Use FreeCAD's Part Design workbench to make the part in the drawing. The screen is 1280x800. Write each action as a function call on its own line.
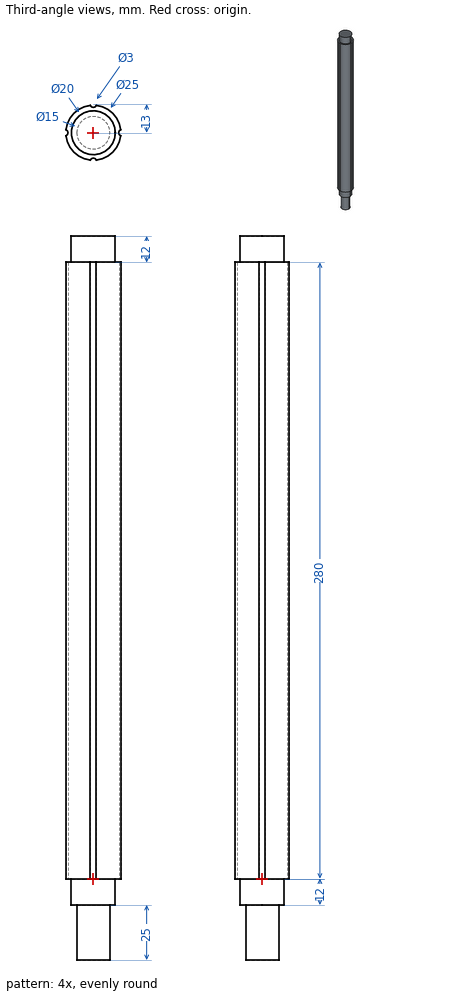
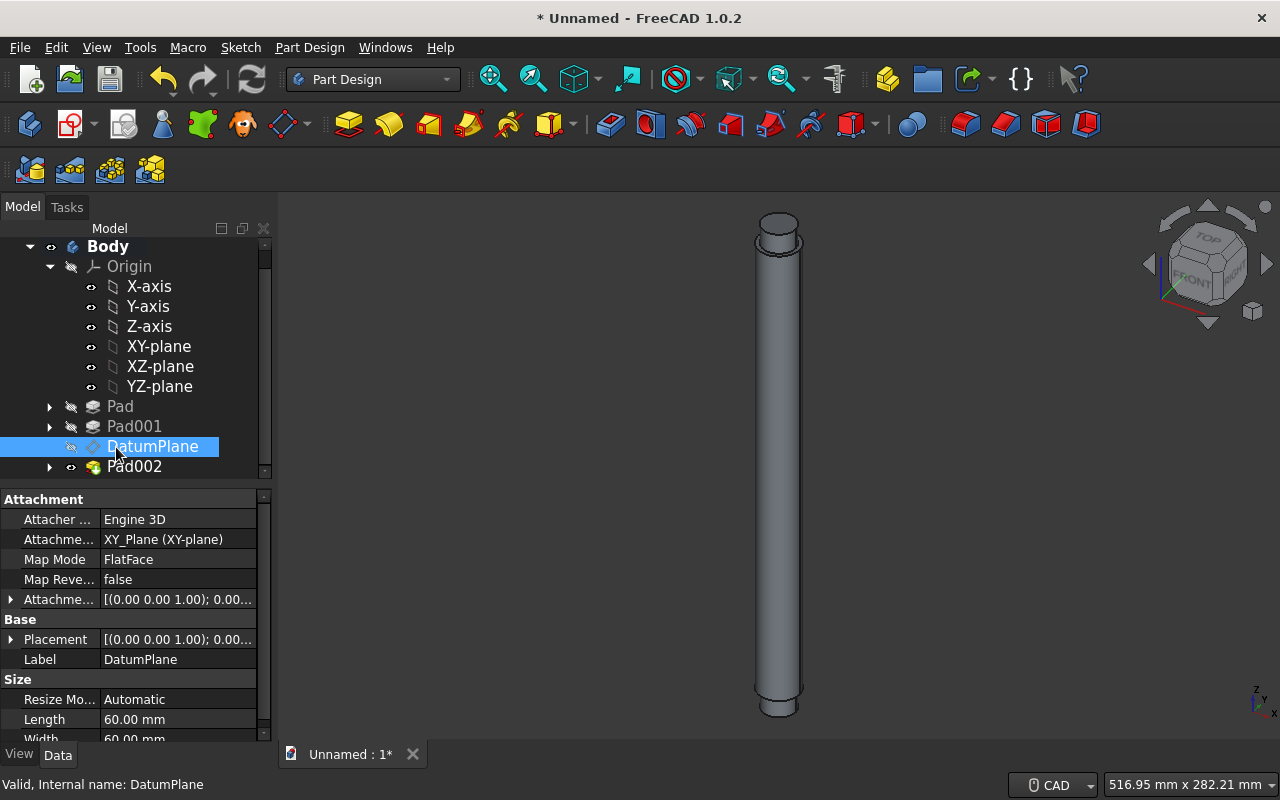
key(5)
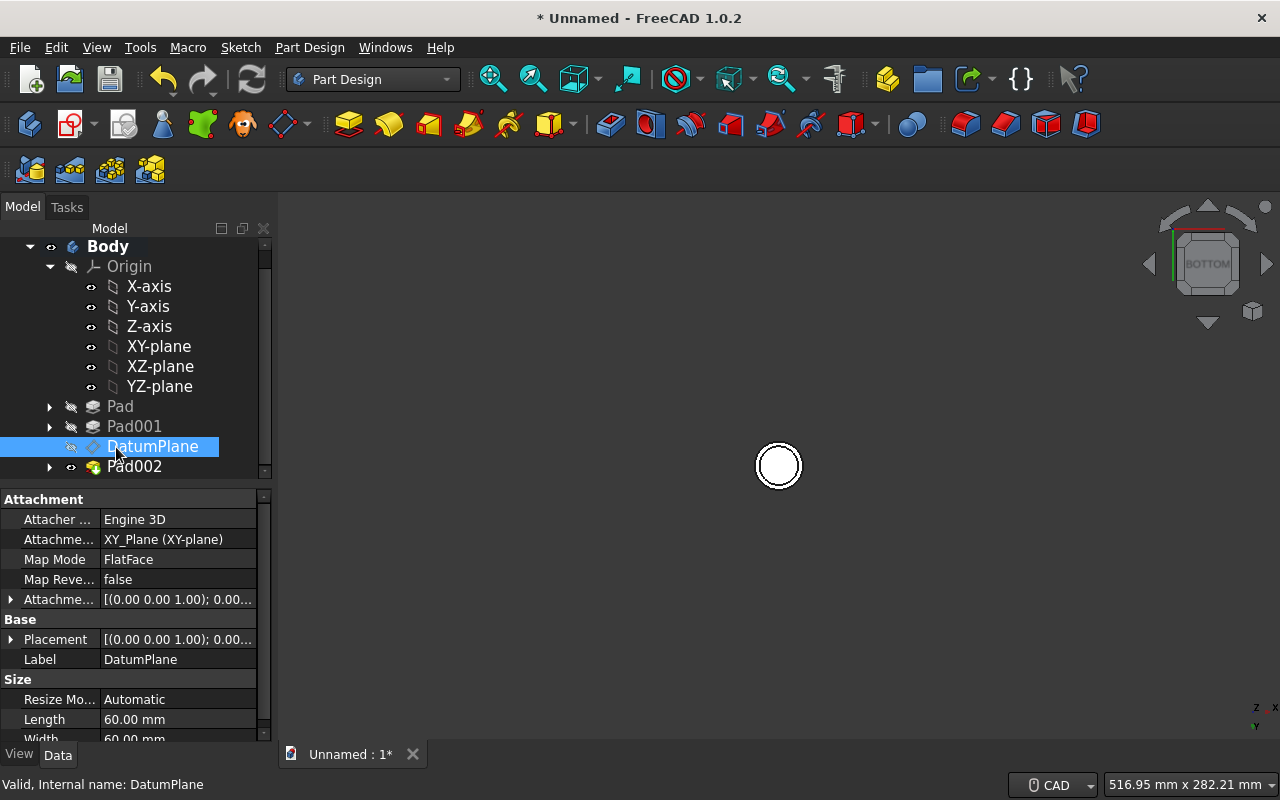
key(v)
key(f)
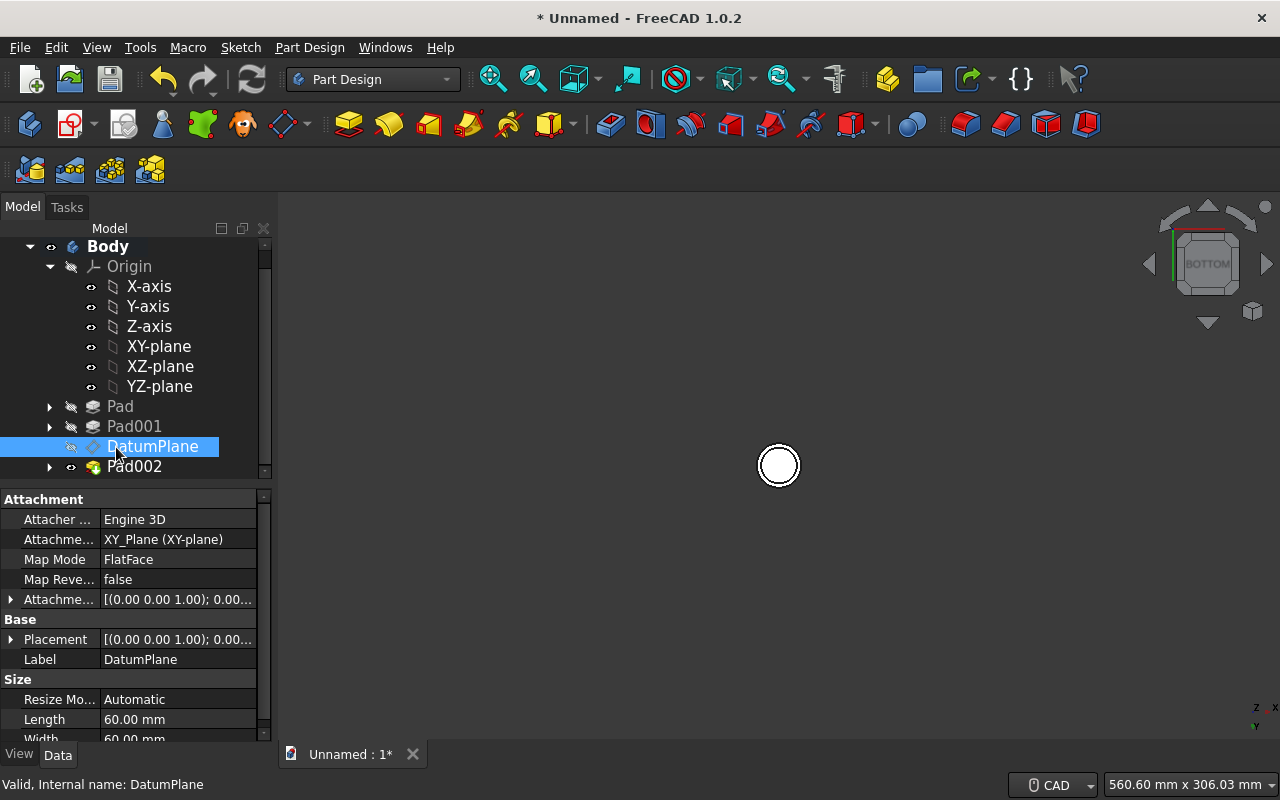
click(779, 464)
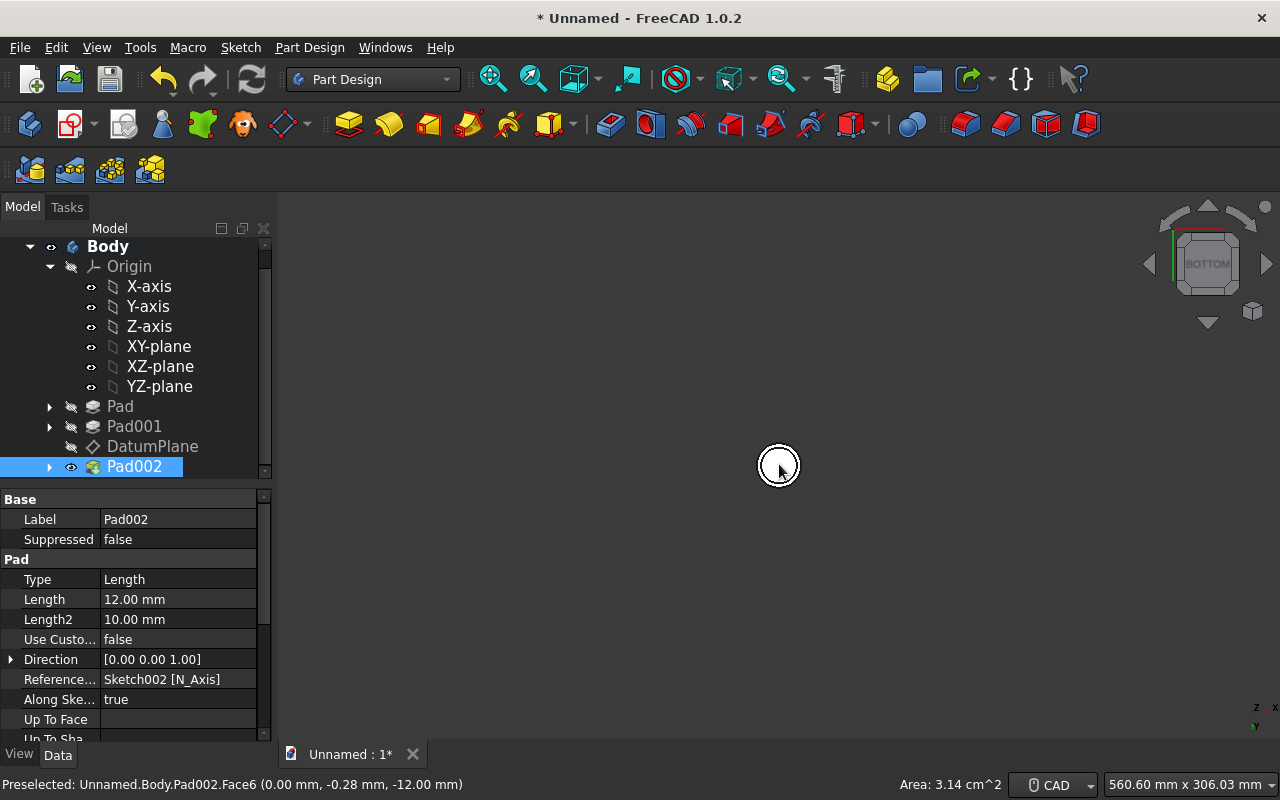
click(70, 124)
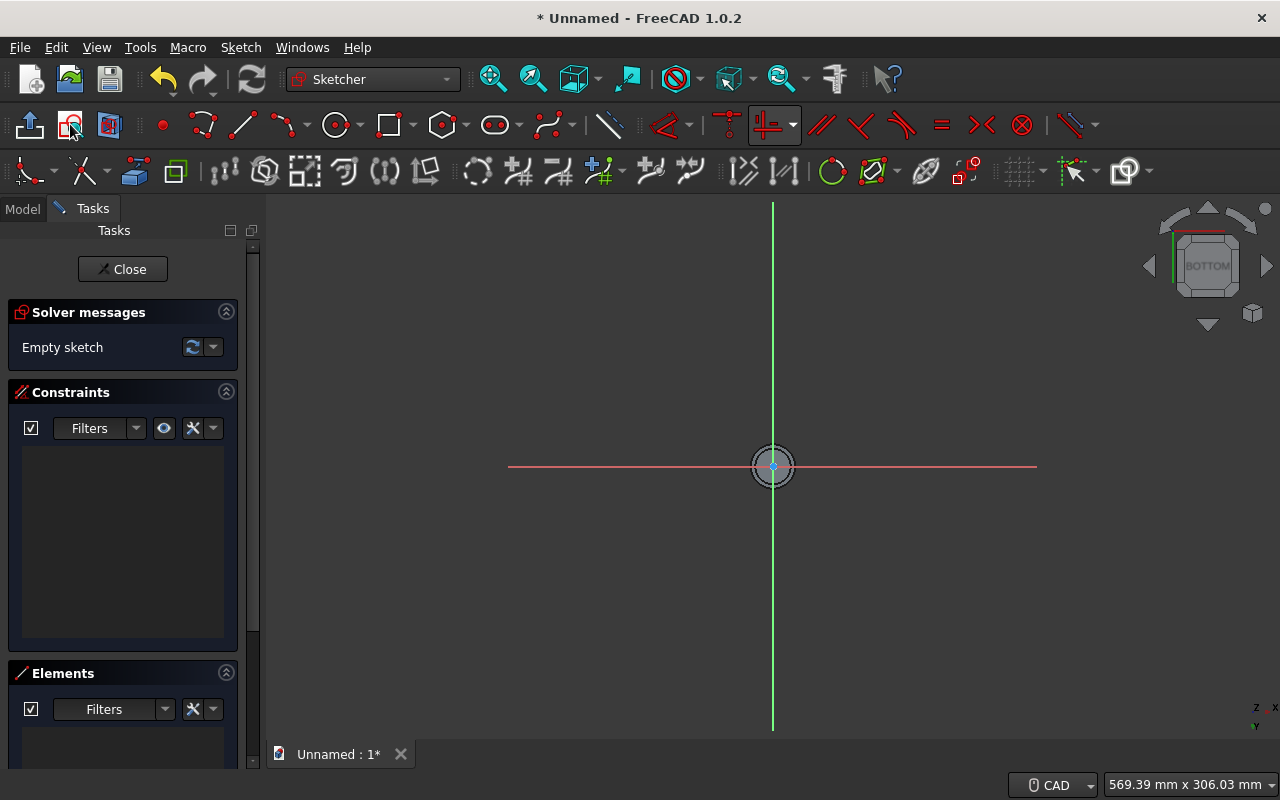
scroll(778, 466, up, 13)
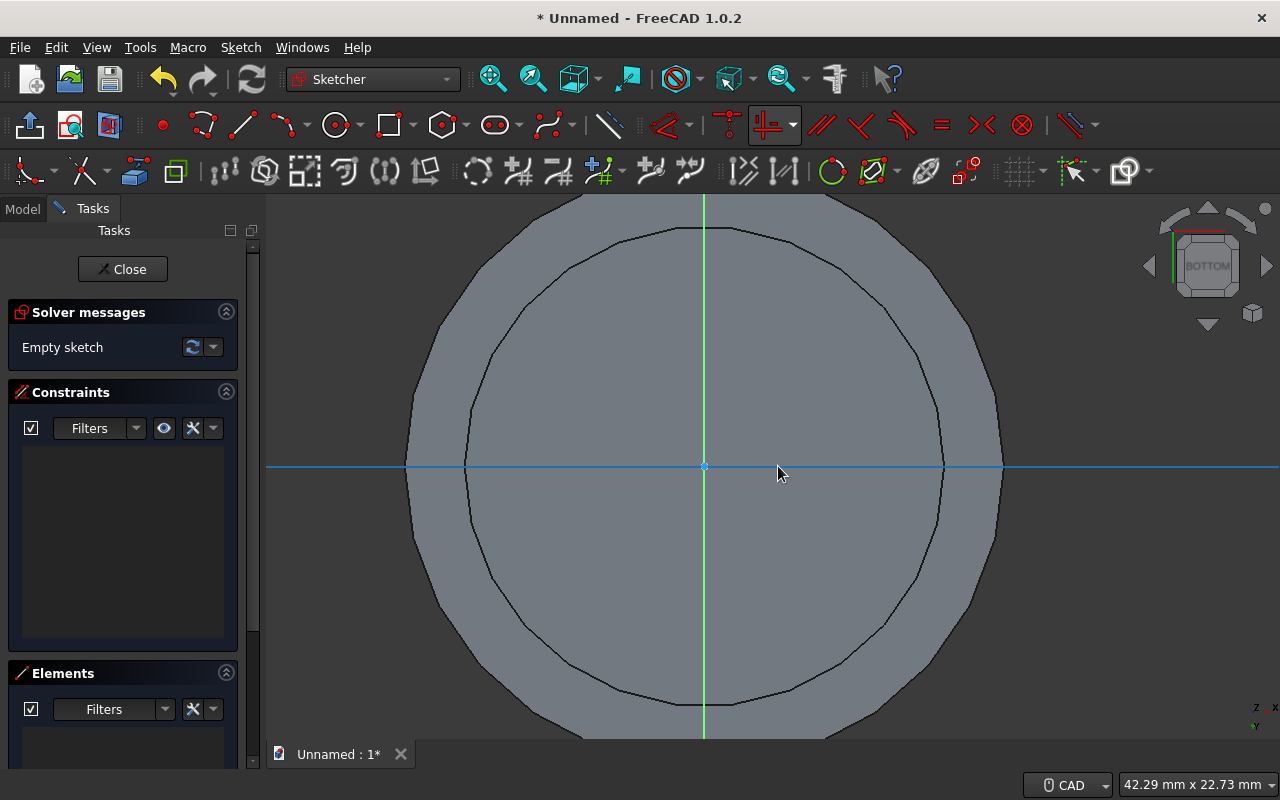
click(336, 126)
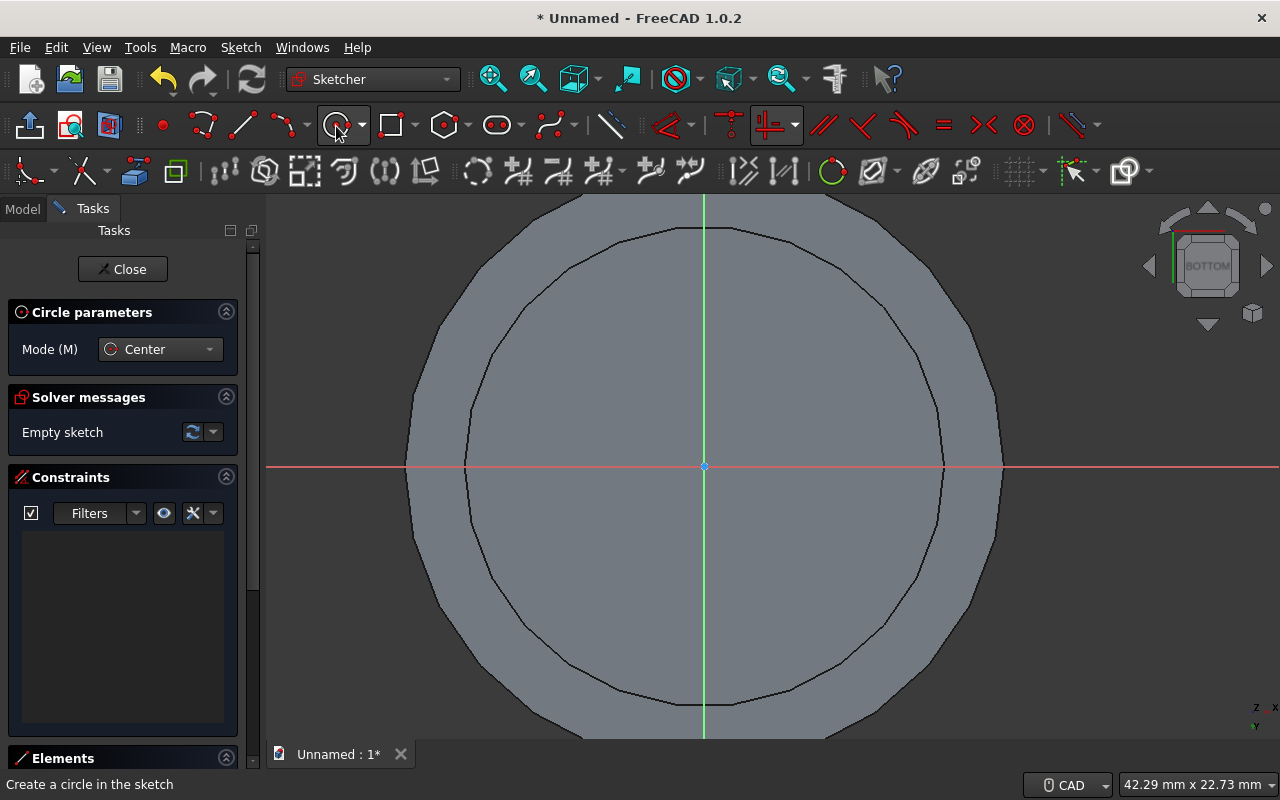
click(704, 466)
click(832, 339)
key(Escape)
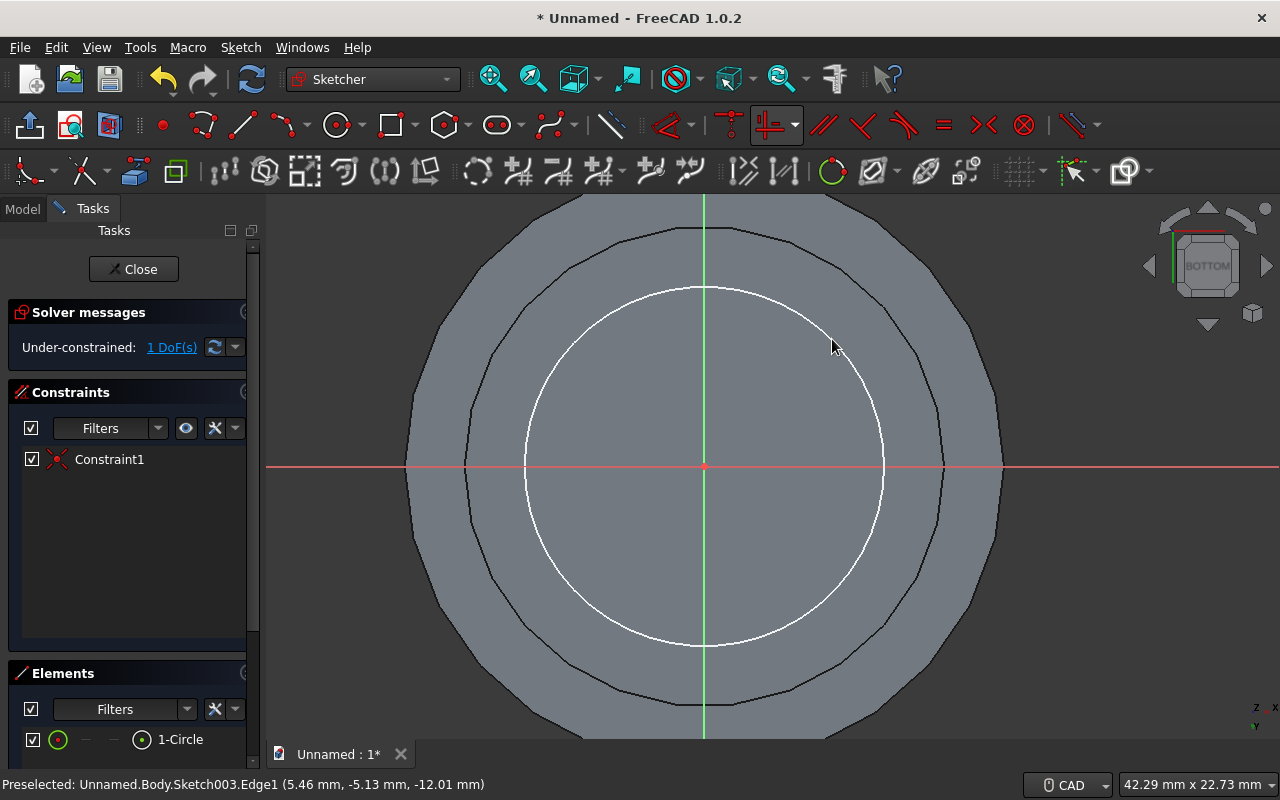
click(666, 126)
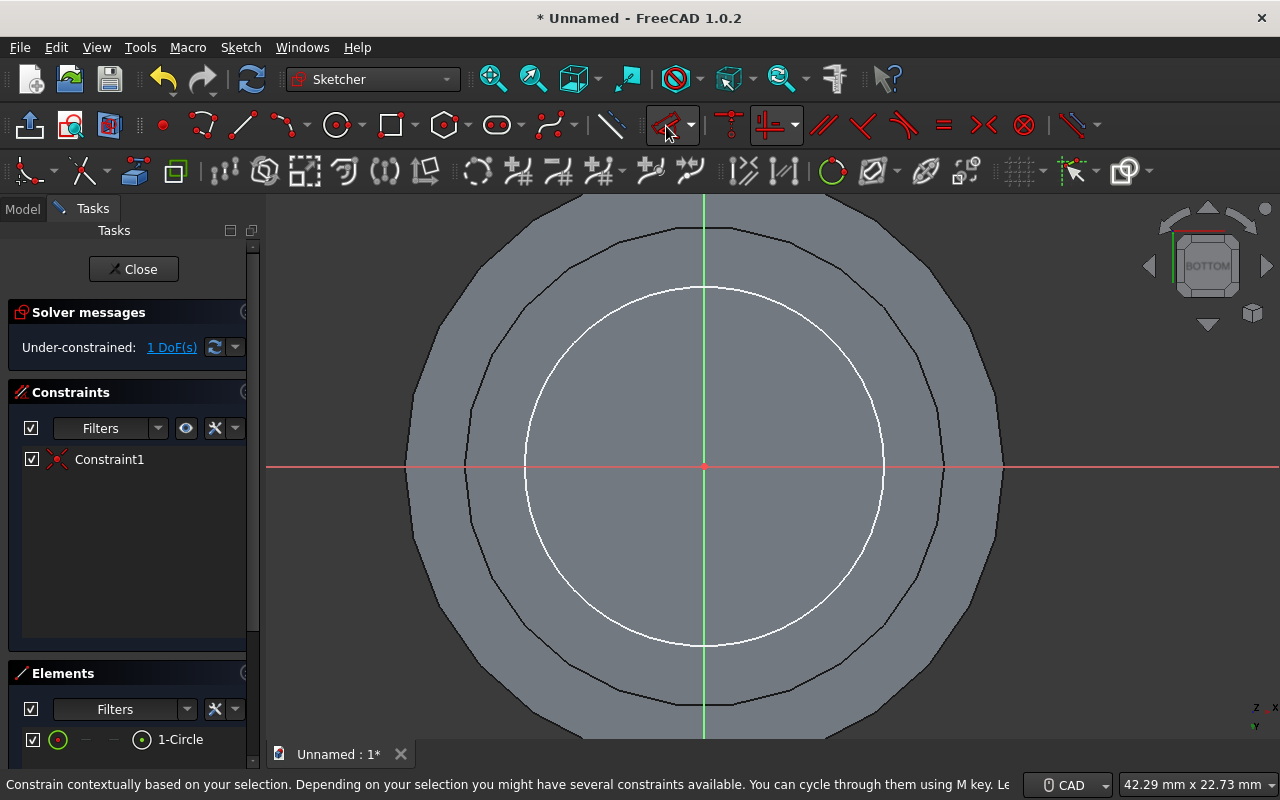
click(831, 339)
click(854, 316)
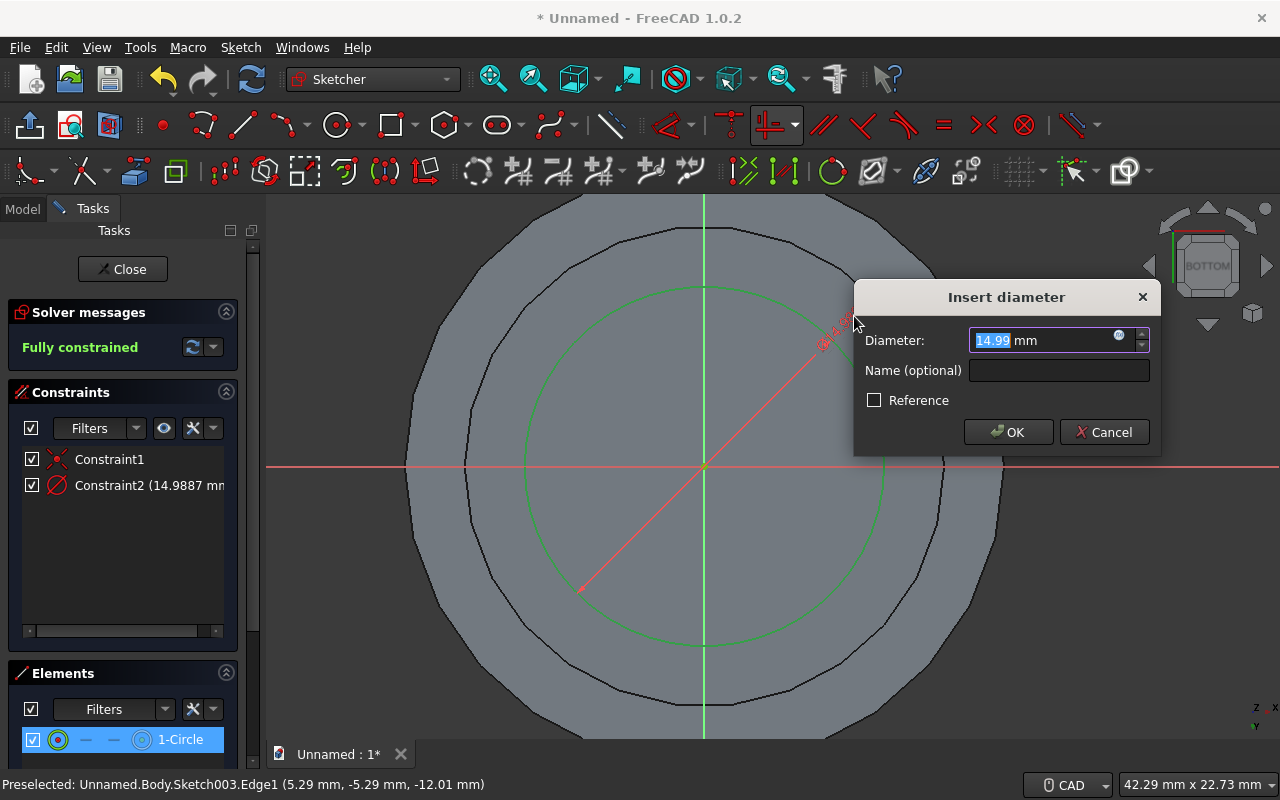
text(15)
key(Return)
key(Escape)